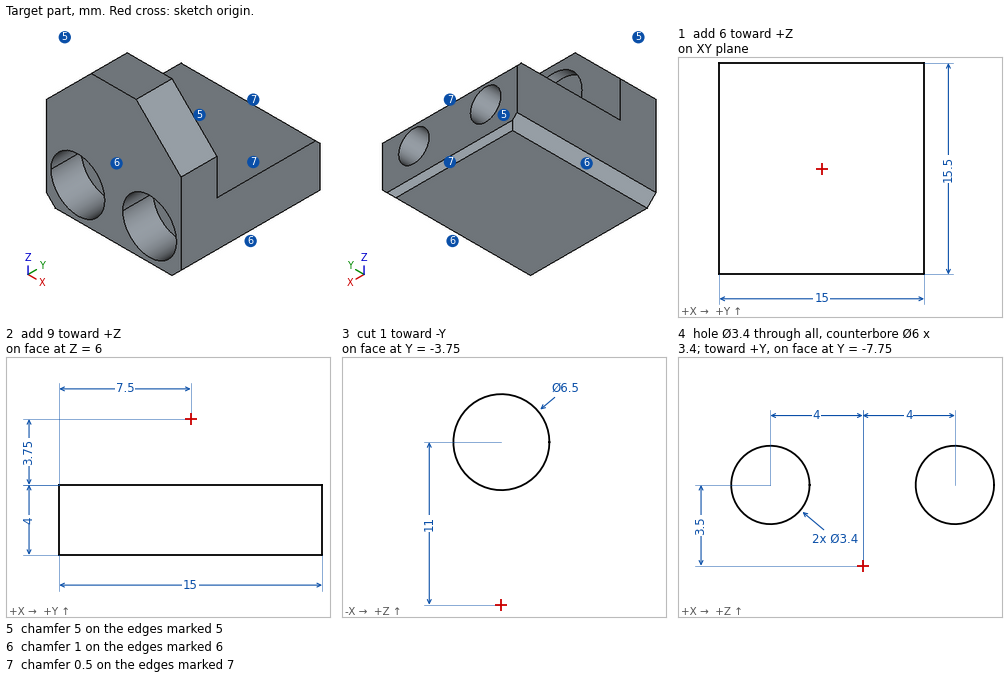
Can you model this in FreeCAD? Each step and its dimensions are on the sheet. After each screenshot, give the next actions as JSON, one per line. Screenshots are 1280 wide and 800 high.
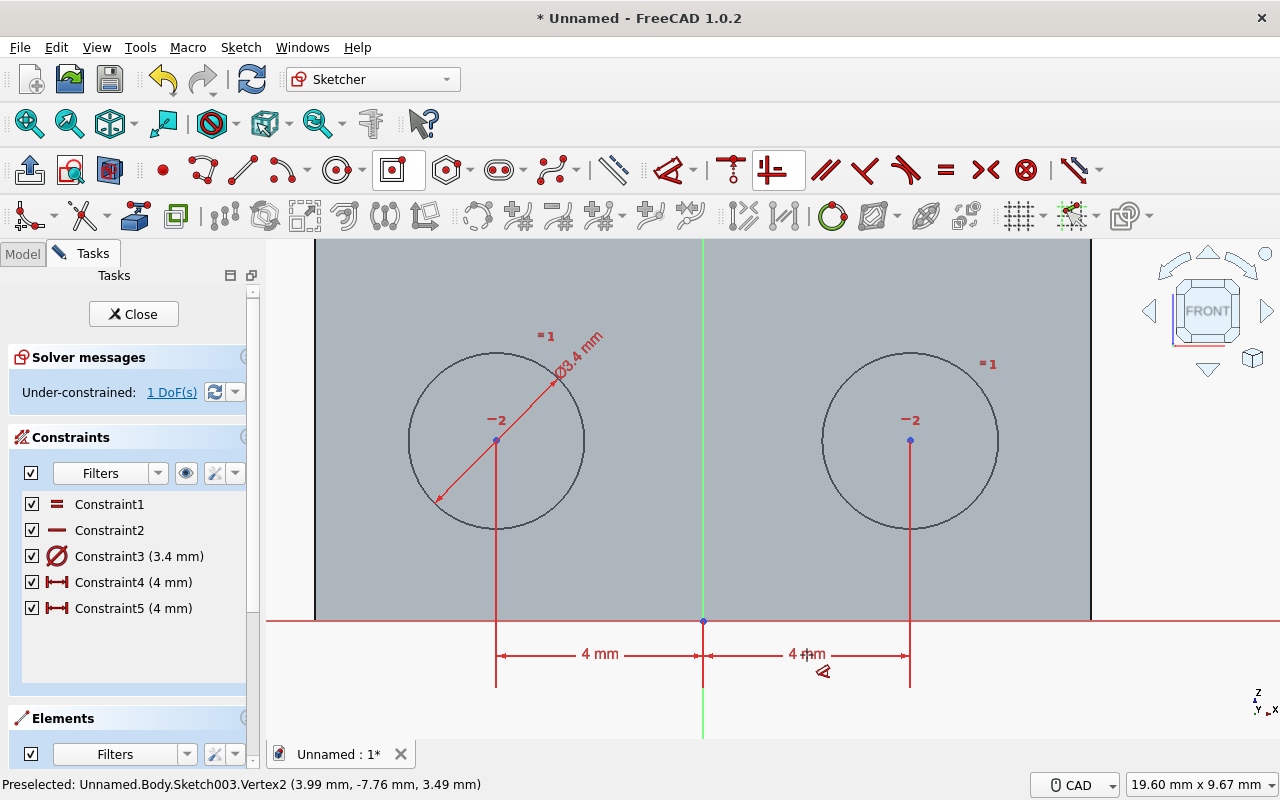
{"action": "left_click", "coordinate": [496, 441]}
{"action": "left_click", "coordinate": [462, 490]}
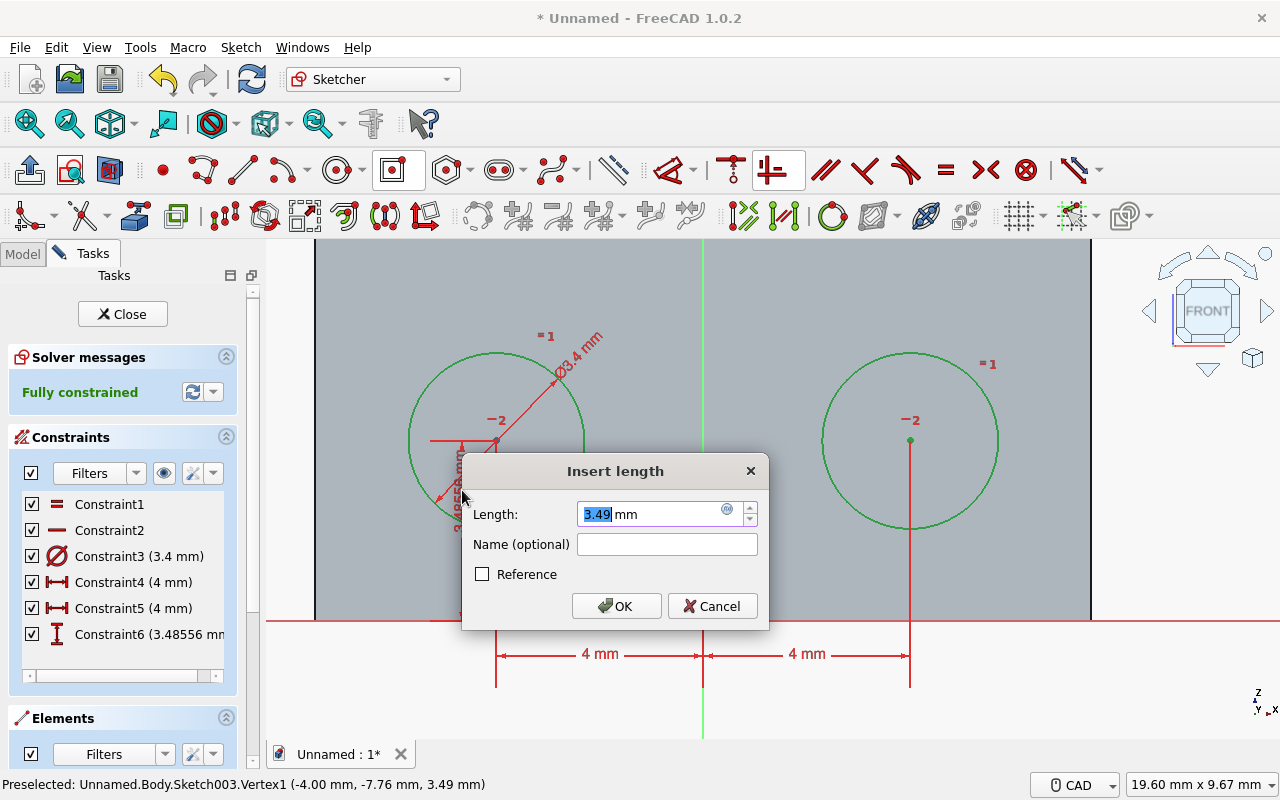
{"action": "type", "text": "3.5"}
{"action": "key", "text": "Return"}
{"action": "key", "text": "Escape"}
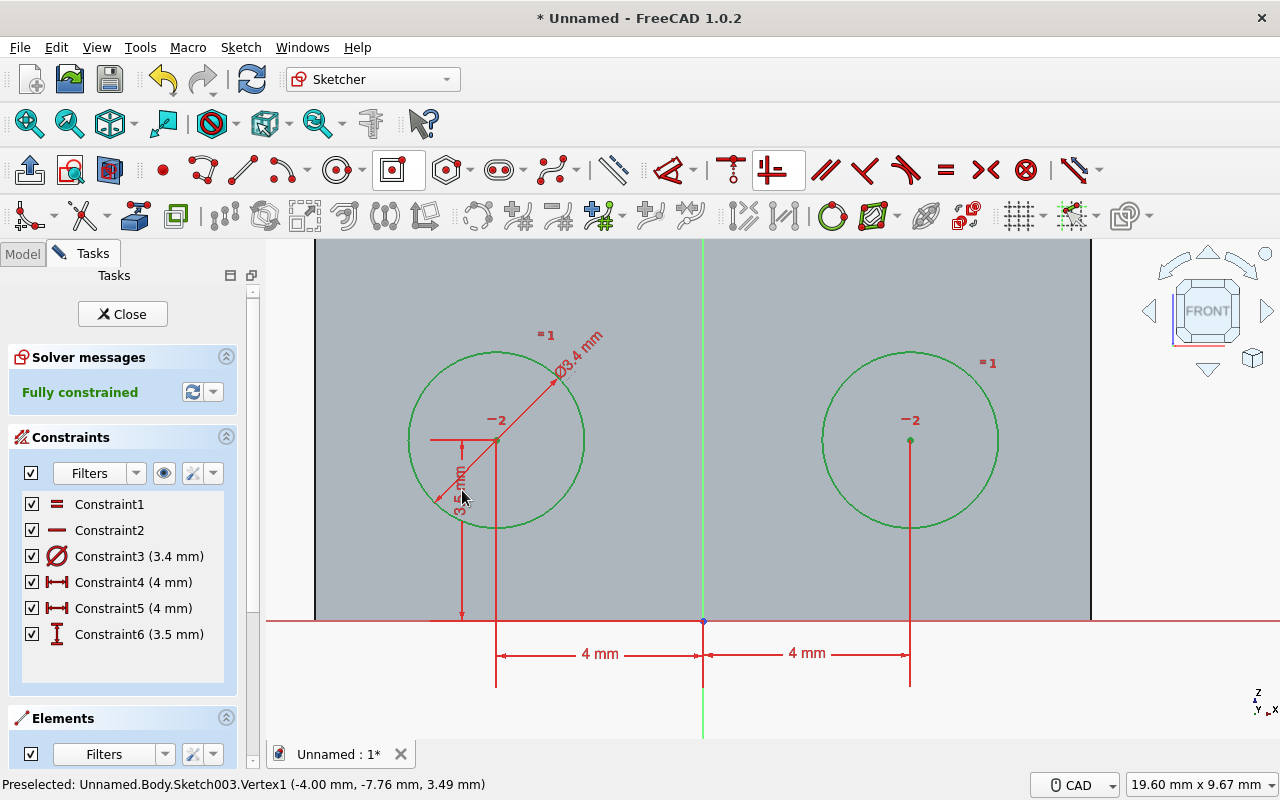
{"action": "left_click", "coordinate": [123, 314]}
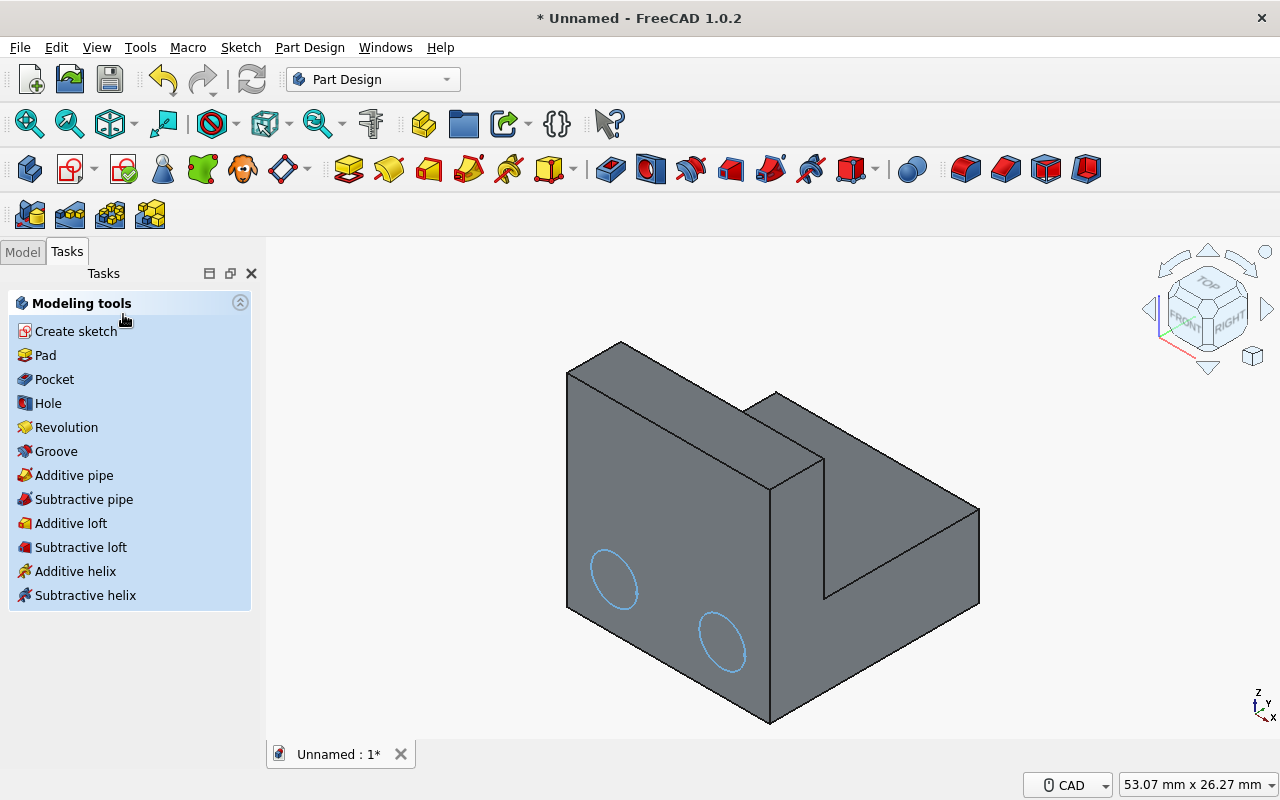
{"action": "left_click", "coordinate": [652, 170]}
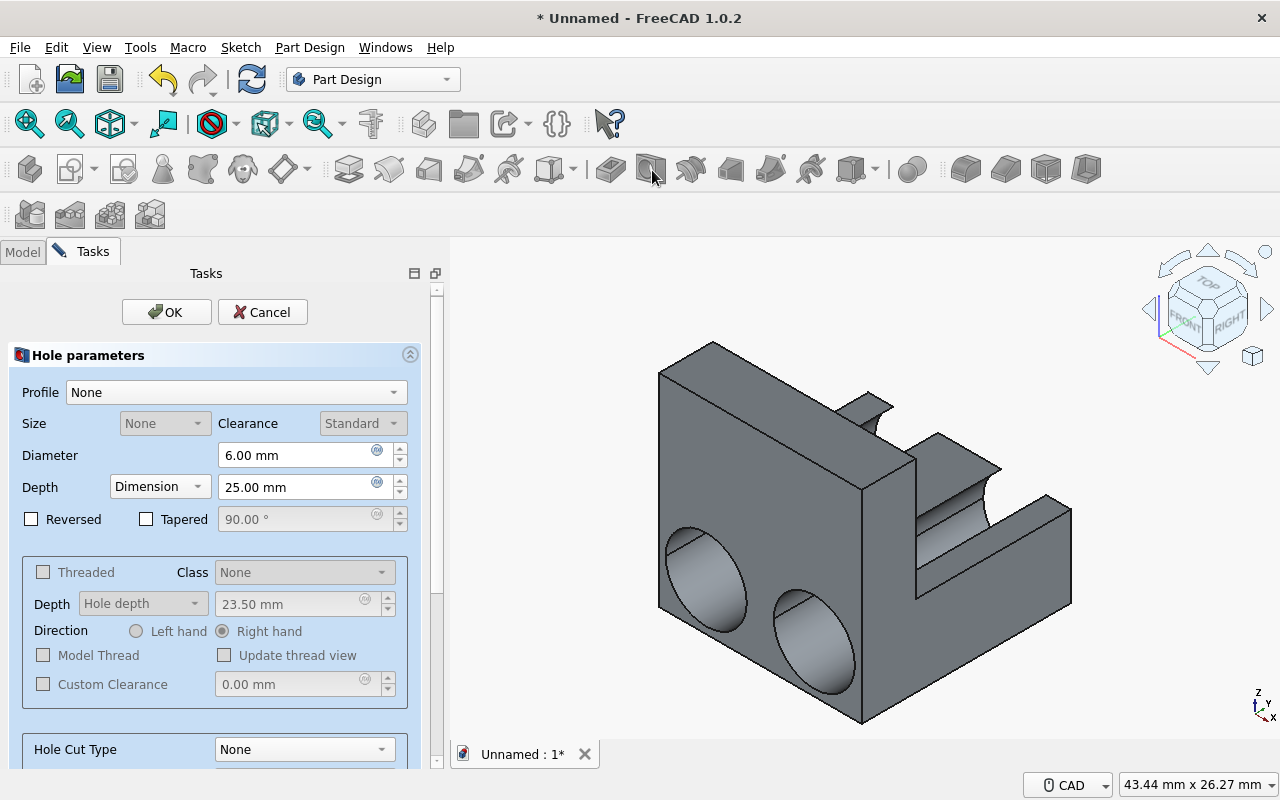
{"action": "triple_click", "coordinate": [305, 455]}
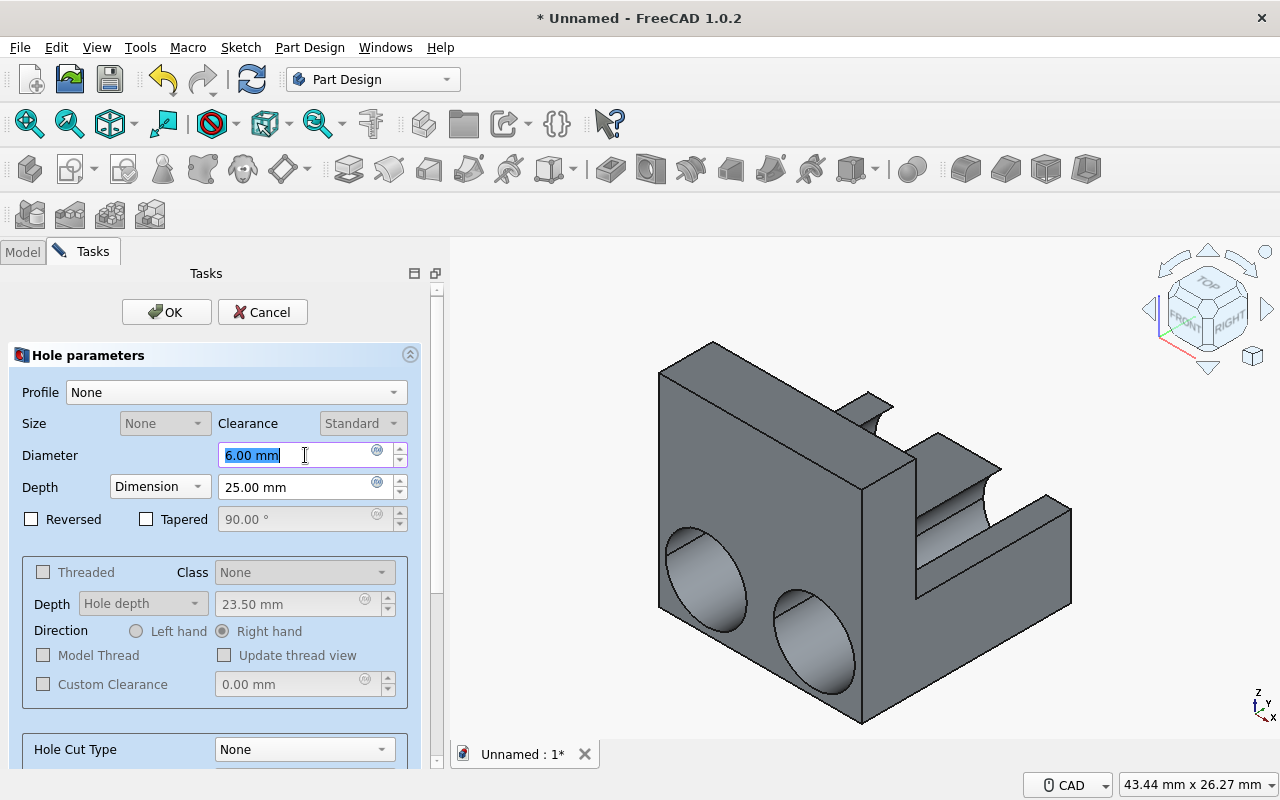
{"action": "type", "text": "3.4"}
{"action": "key", "text": "Tab"}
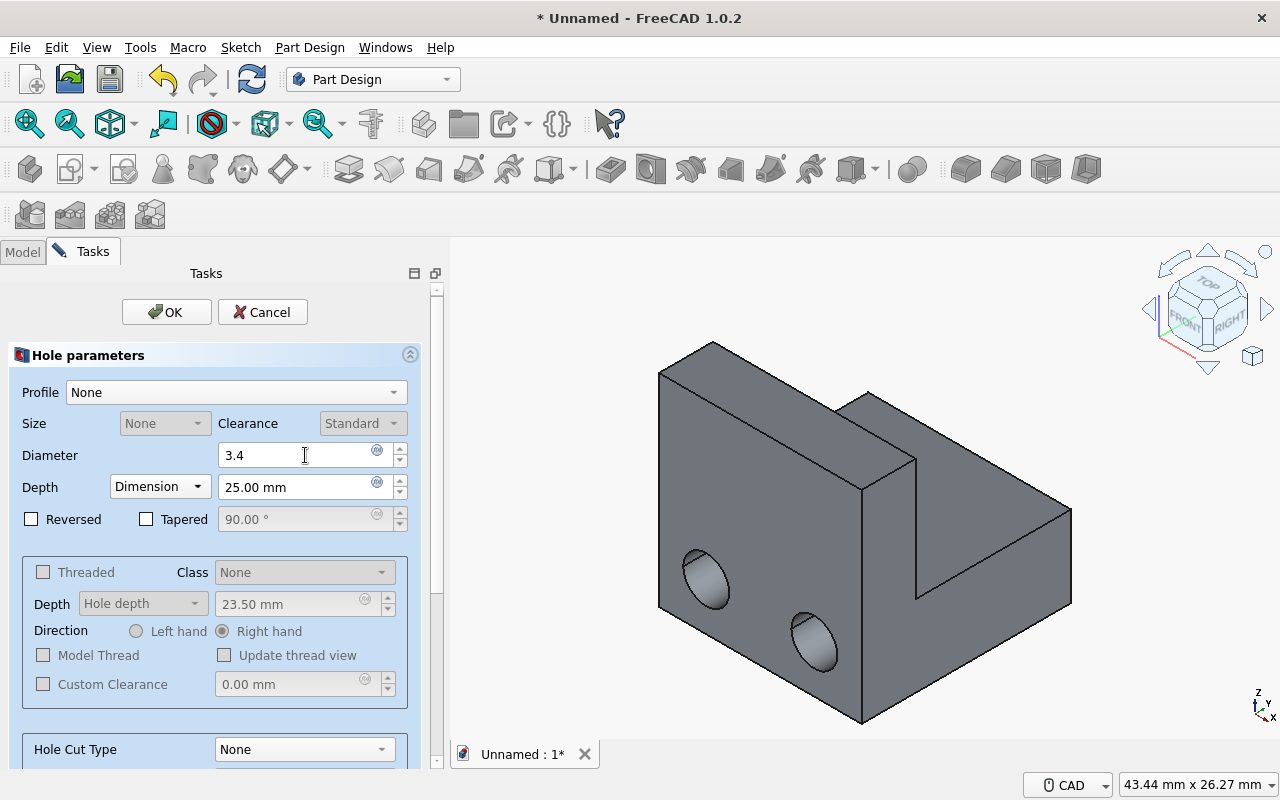
{"action": "left_click", "coordinate": [161, 486]}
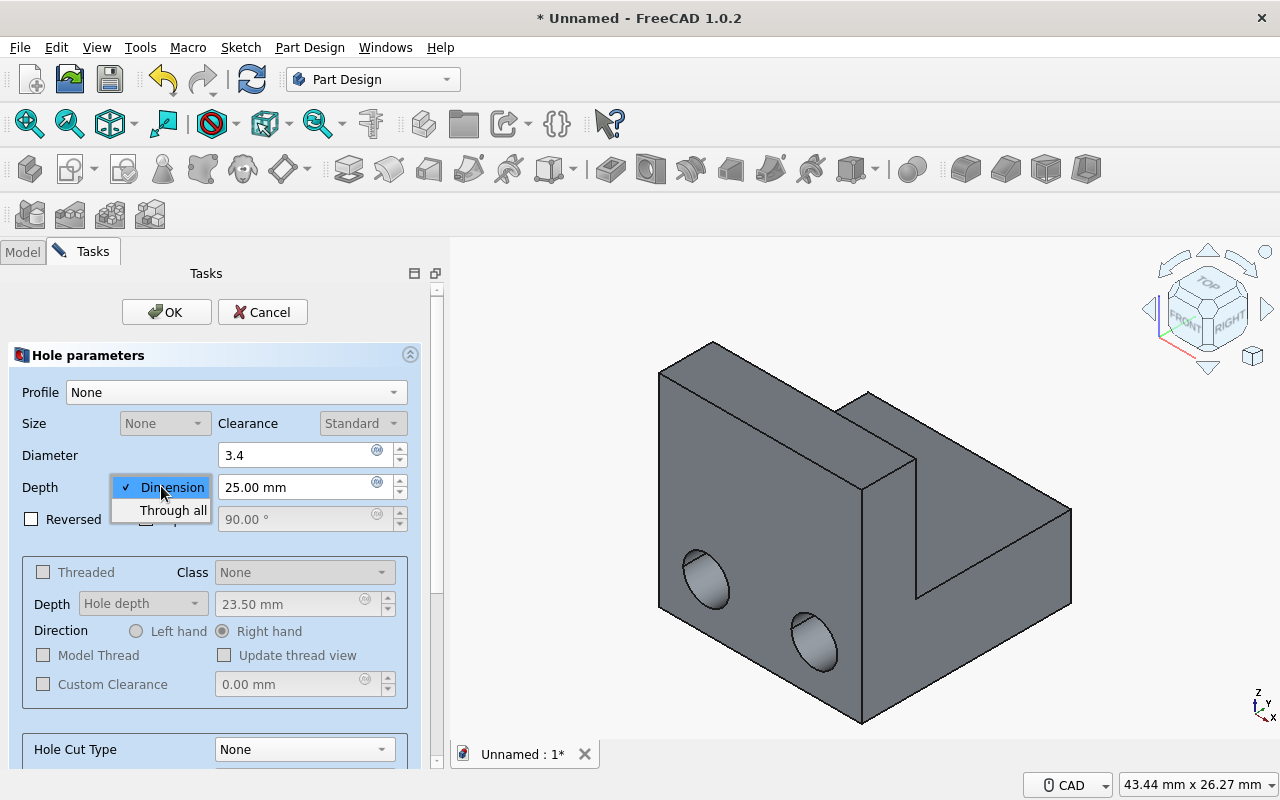
{"action": "left_click", "coordinate": [160, 510]}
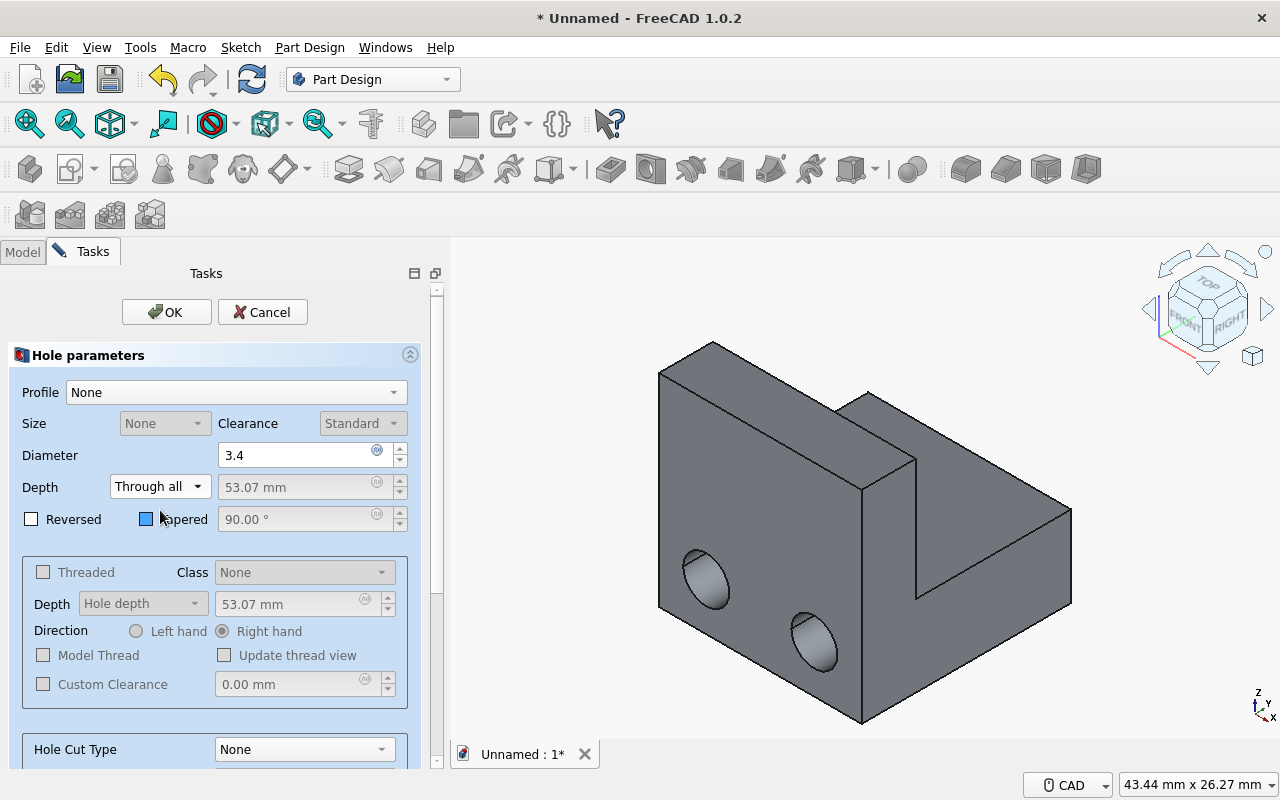
{"action": "left_click", "coordinate": [306, 750]}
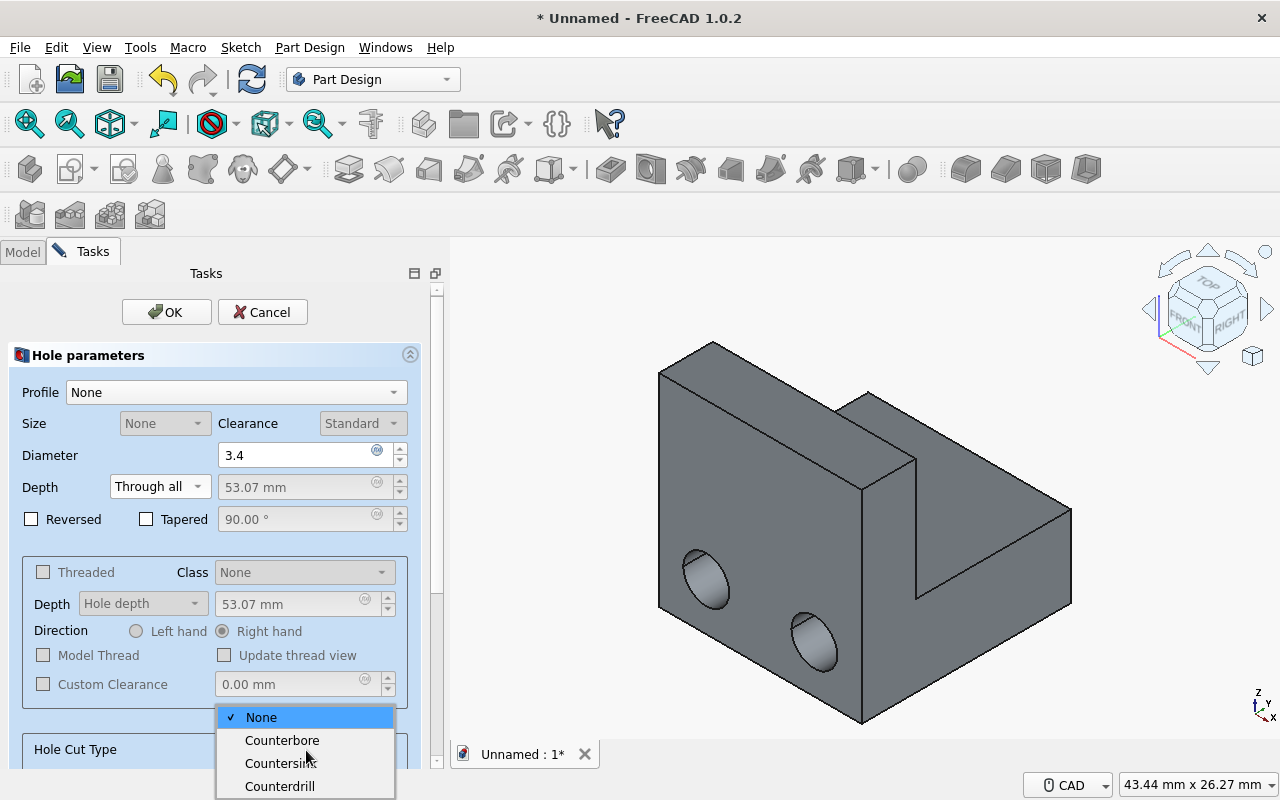
{"action": "left_click", "coordinate": [304, 740]}